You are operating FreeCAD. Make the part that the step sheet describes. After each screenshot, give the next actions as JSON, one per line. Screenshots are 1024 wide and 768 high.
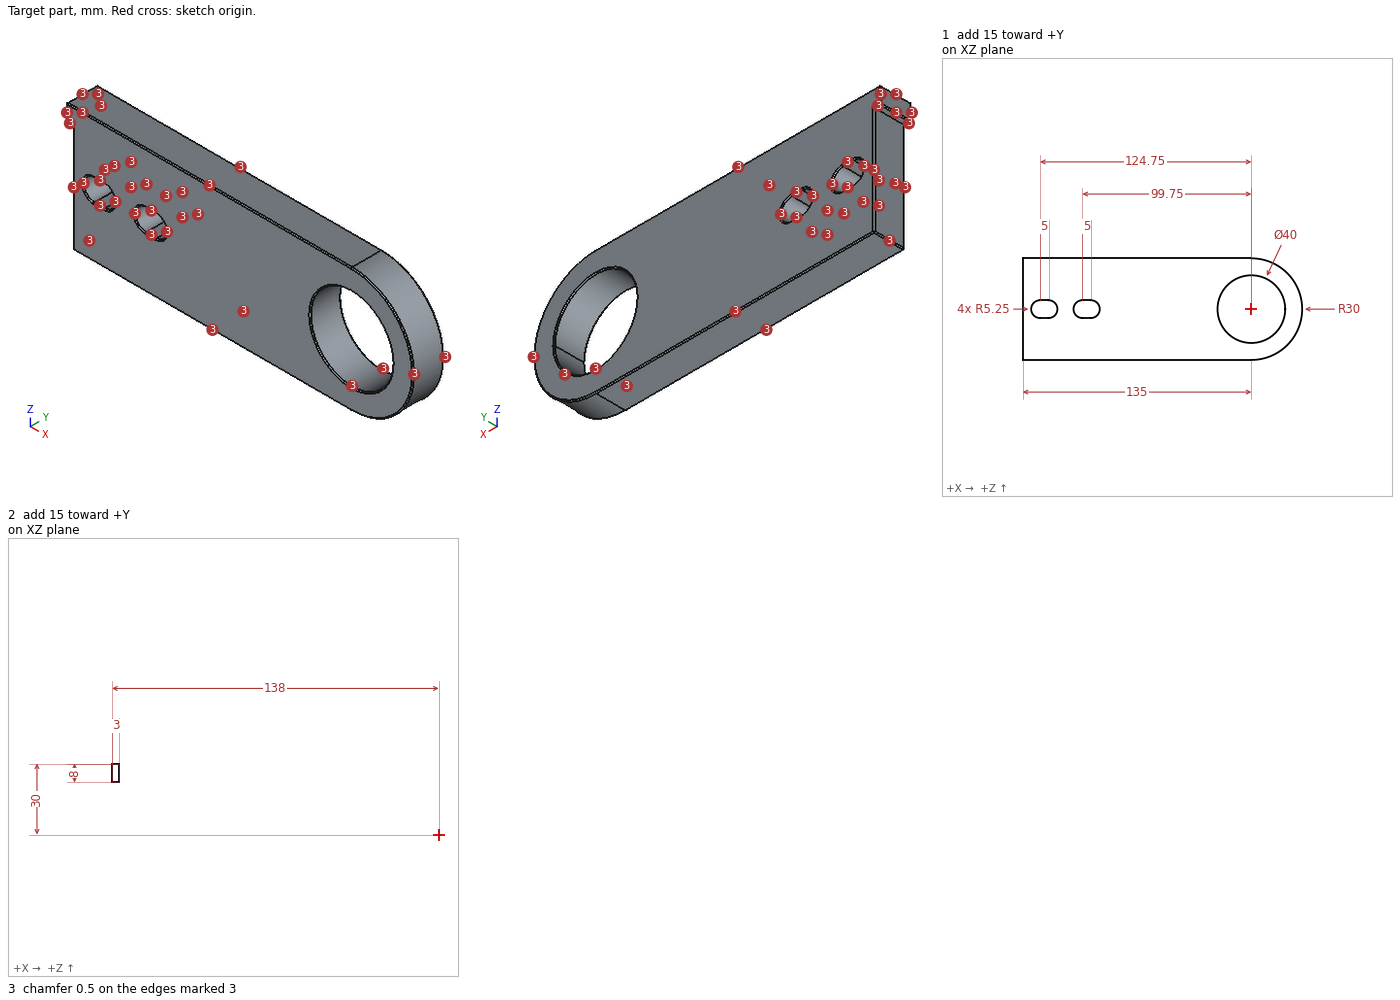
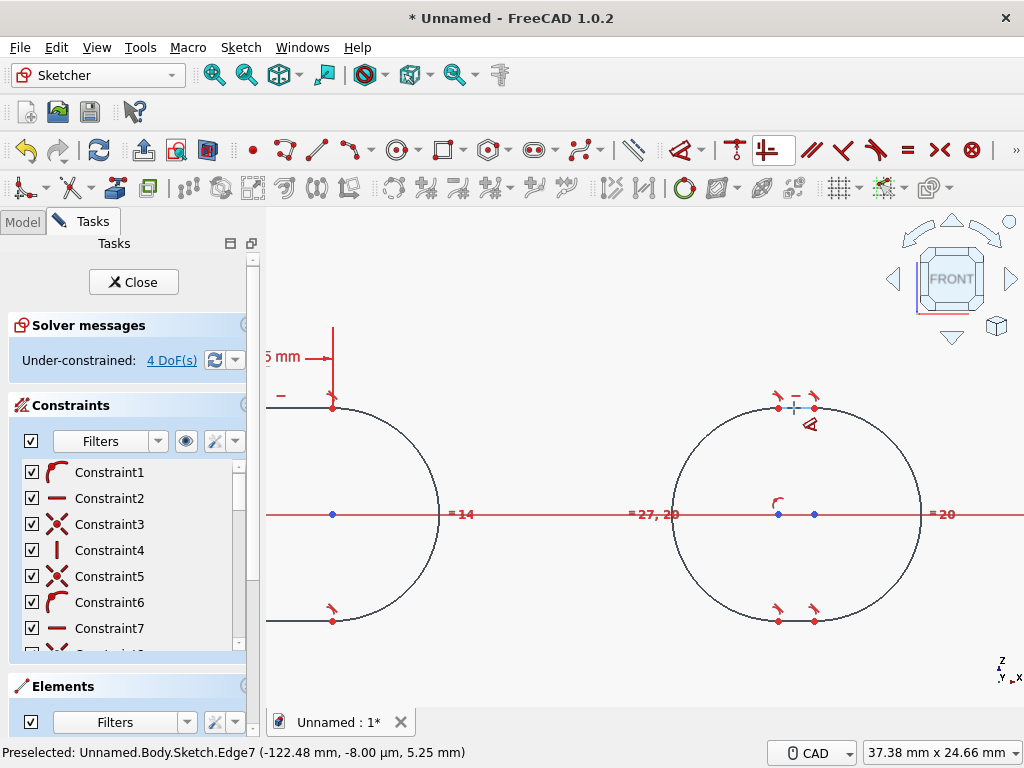
{"action": "left_click", "coordinate": [793, 408]}
{"action": "left_click", "coordinate": [797, 374]}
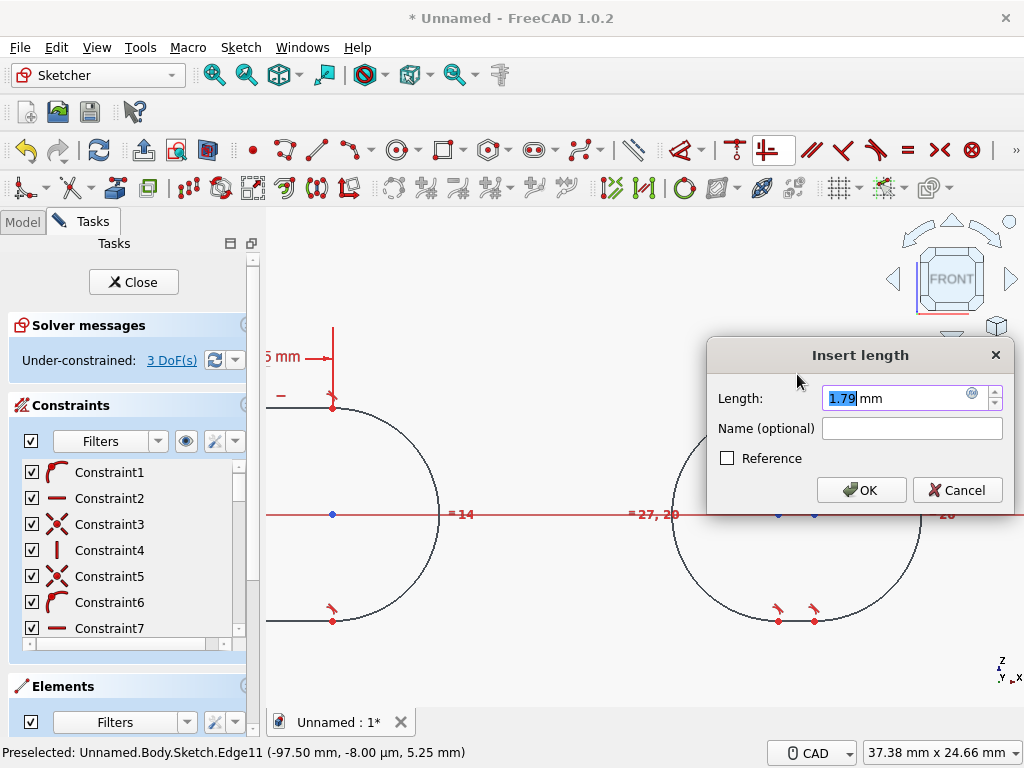
{"action": "type", "text": "5"}
{"action": "key", "text": "Return"}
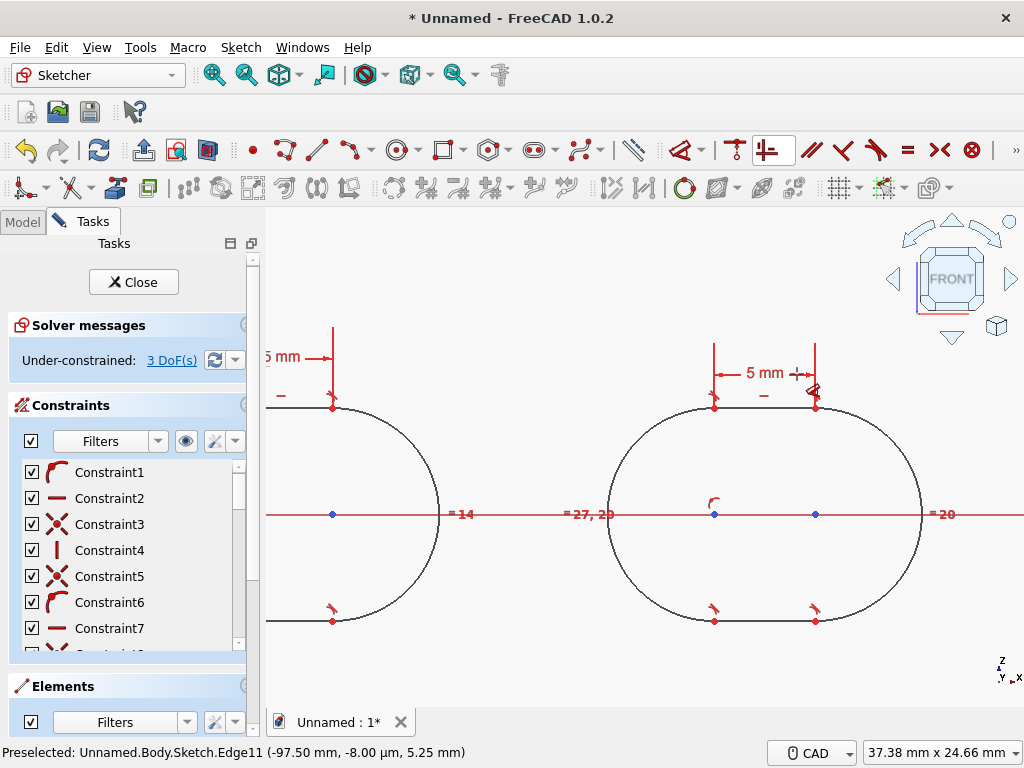
{"action": "scroll", "coordinate": [436, 450], "scroll_direction": "down", "scroll_amount": 11}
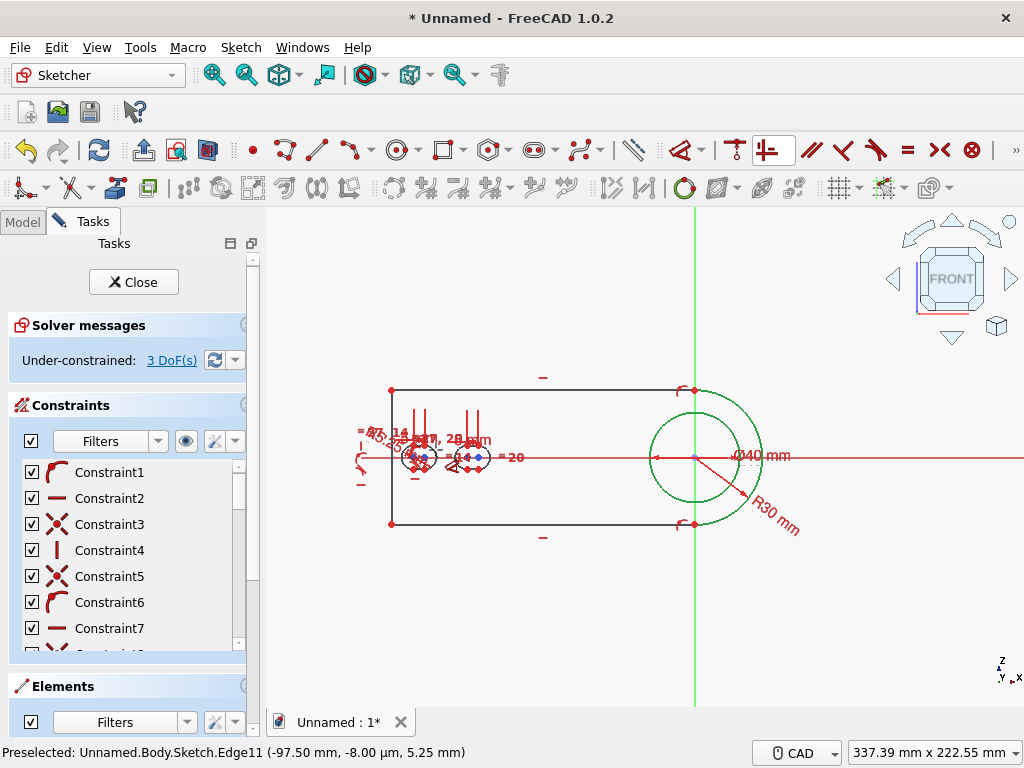
{"action": "left_click", "coordinate": [604, 525]}
{"action": "left_click", "coordinate": [543, 559]}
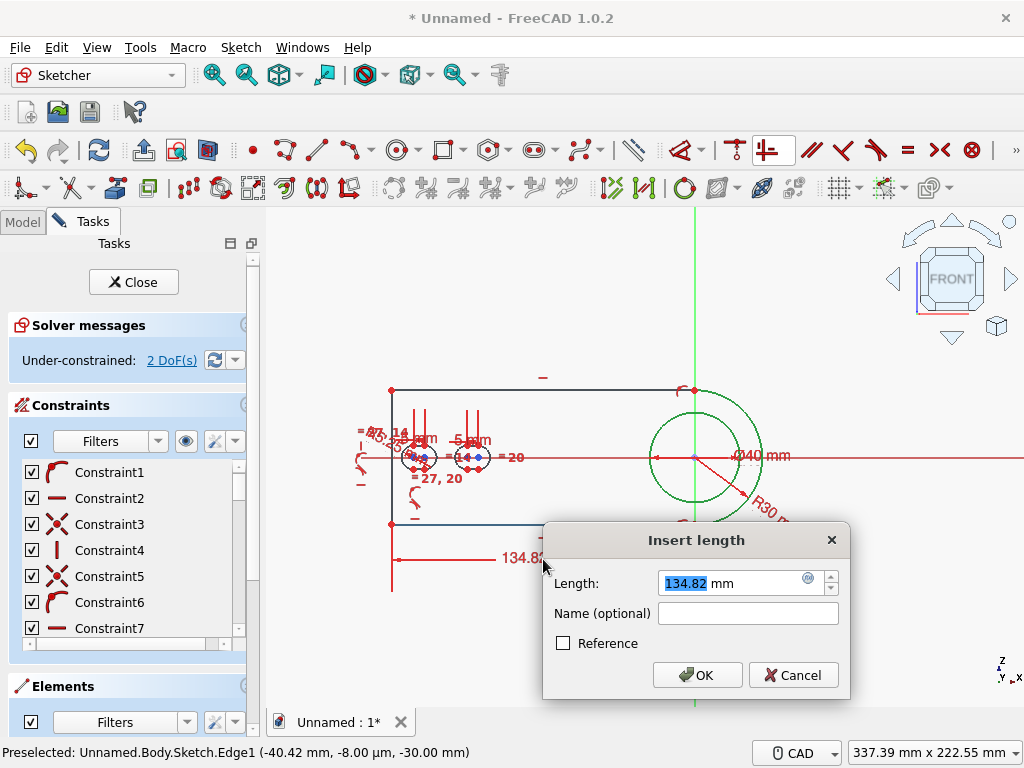
{"action": "type", "text": "135"}
{"action": "key", "text": "Return"}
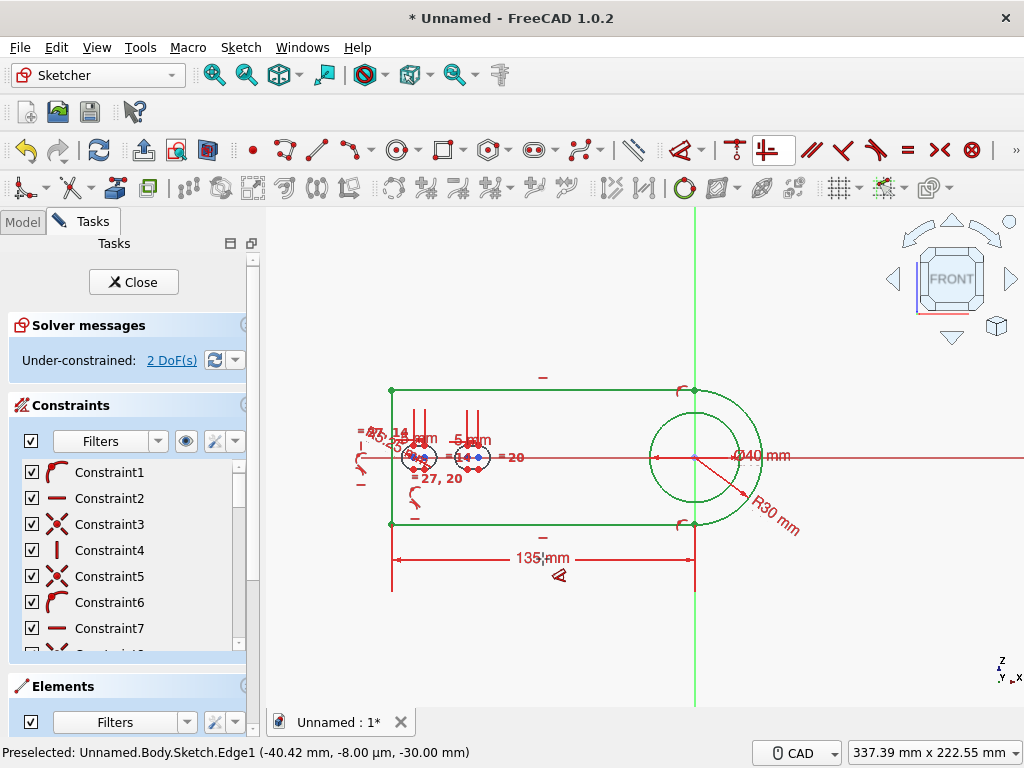
{"action": "left_click", "coordinate": [467, 446]}
{"action": "left_click", "coordinate": [581, 412]}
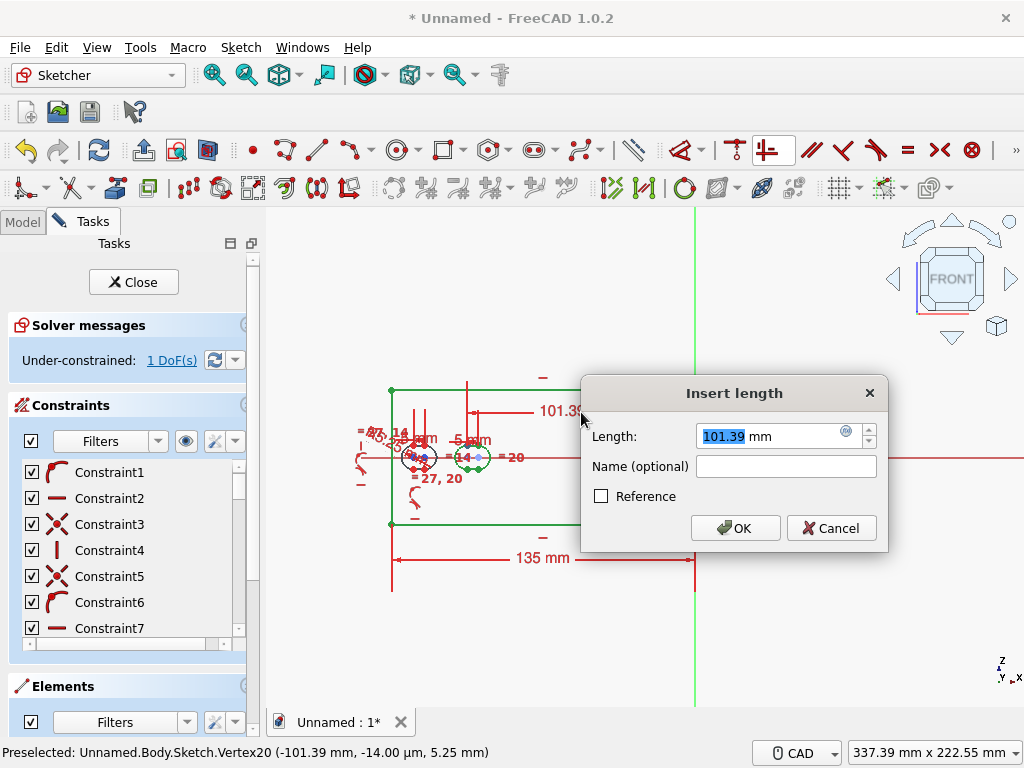
{"action": "type", "text": "99.75"}
{"action": "key", "text": "Return"}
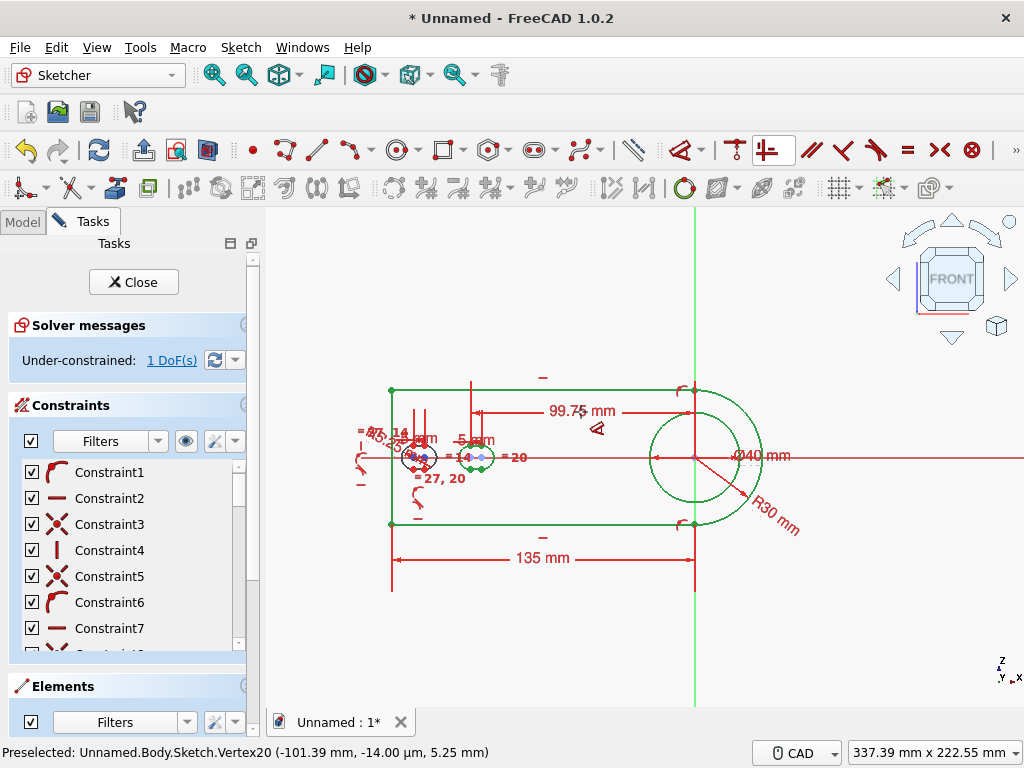
{"action": "left_click", "coordinate": [414, 446]}
{"action": "left_click", "coordinate": [489, 412]}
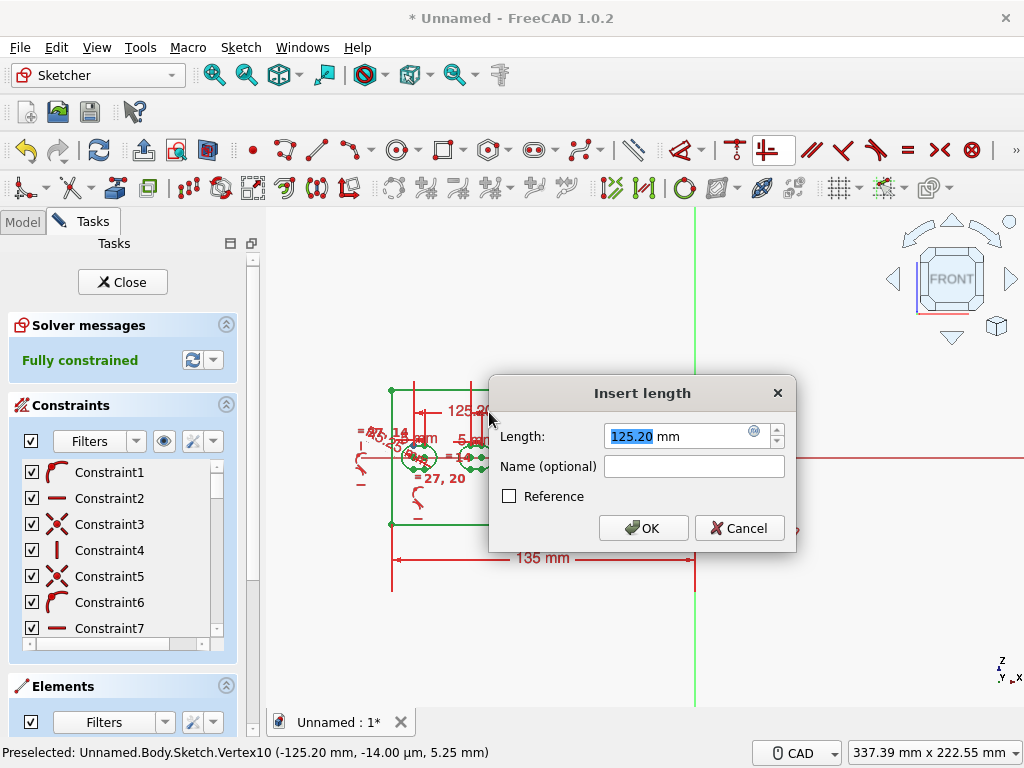
{"action": "type", "text": "124.75"}
{"action": "key", "text": "Return"}
{"action": "key", "text": "Escape"}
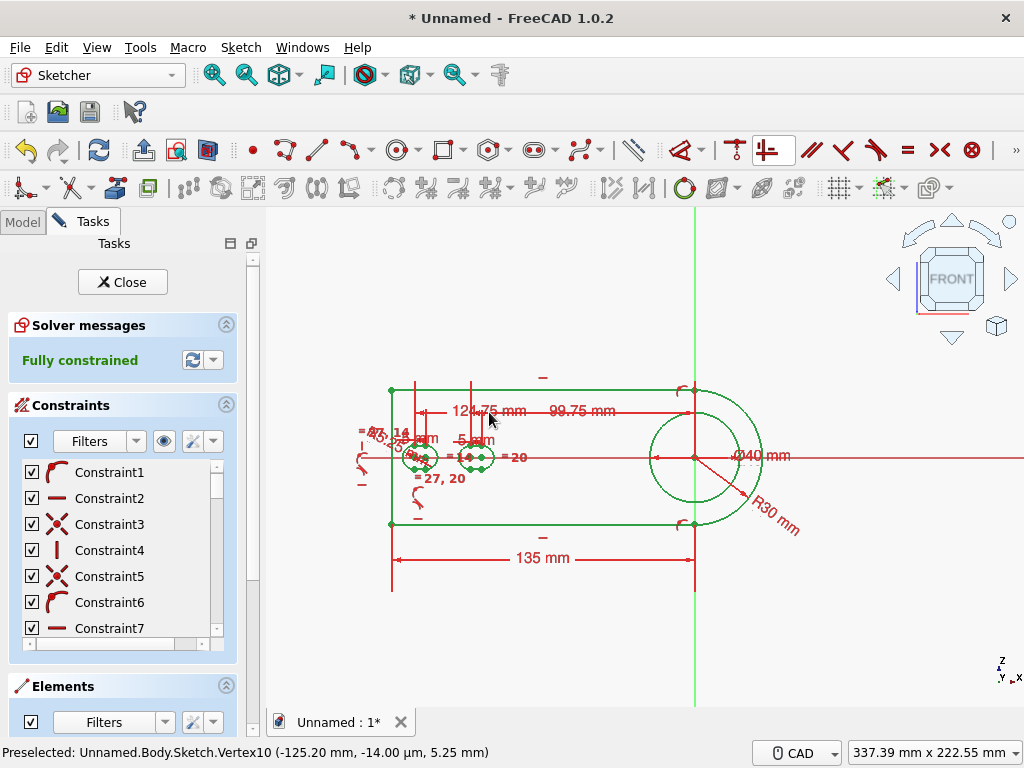
{"action": "left_click", "coordinate": [123, 282]}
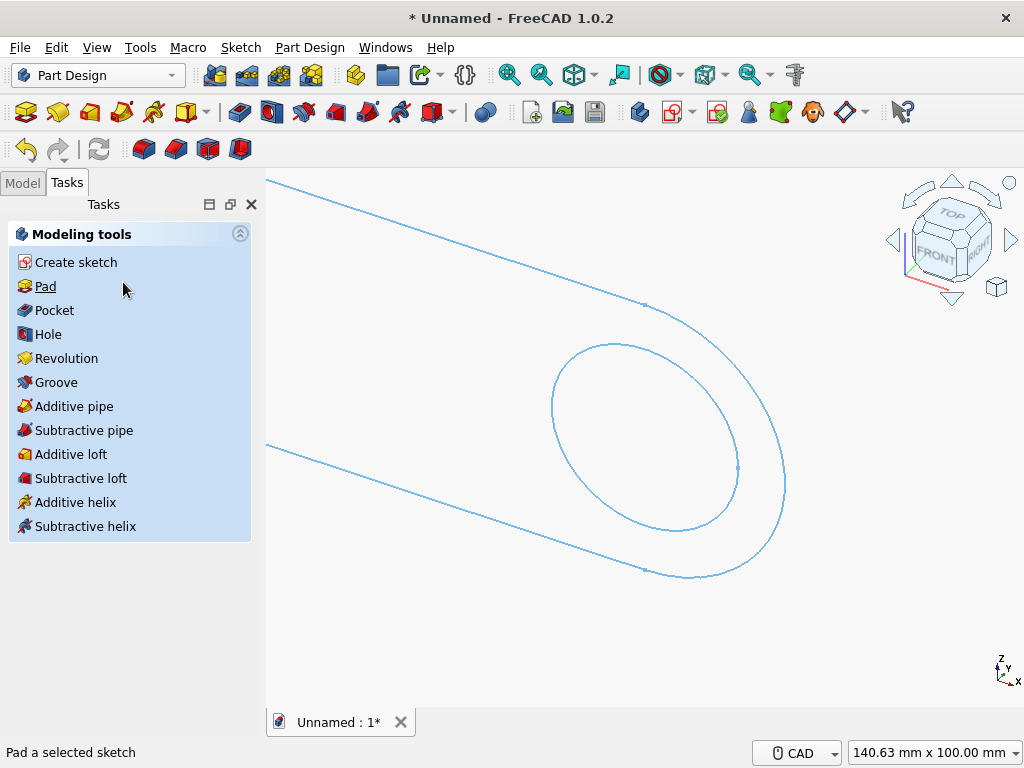
{"action": "left_click", "coordinate": [26, 112]}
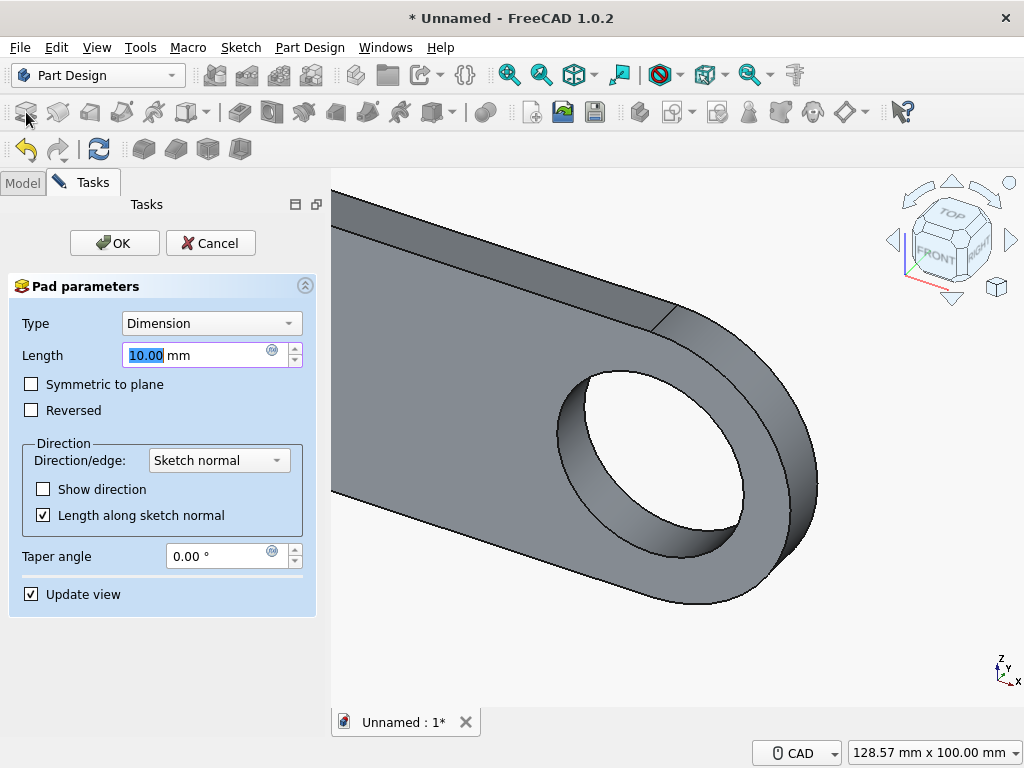
{"action": "type", "text": "15"}
{"action": "key", "text": "Tab"}